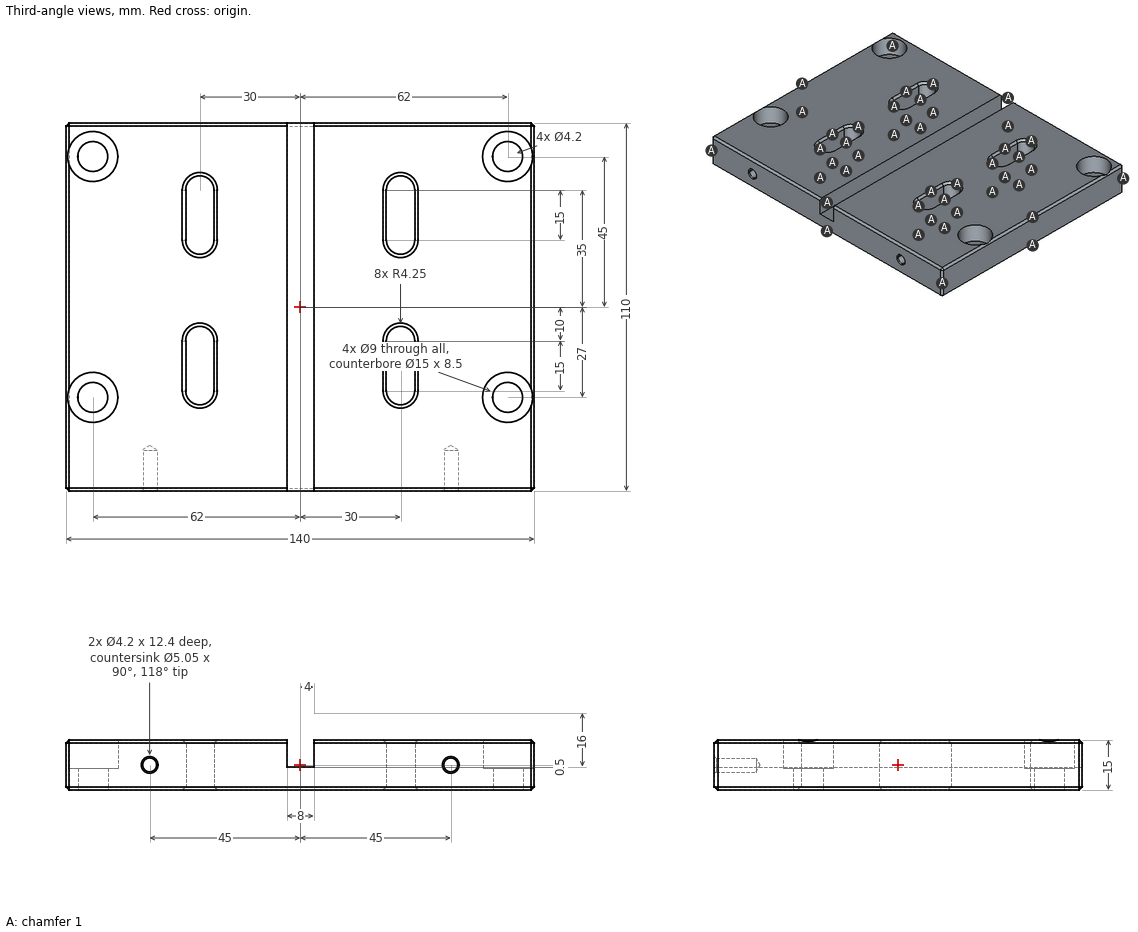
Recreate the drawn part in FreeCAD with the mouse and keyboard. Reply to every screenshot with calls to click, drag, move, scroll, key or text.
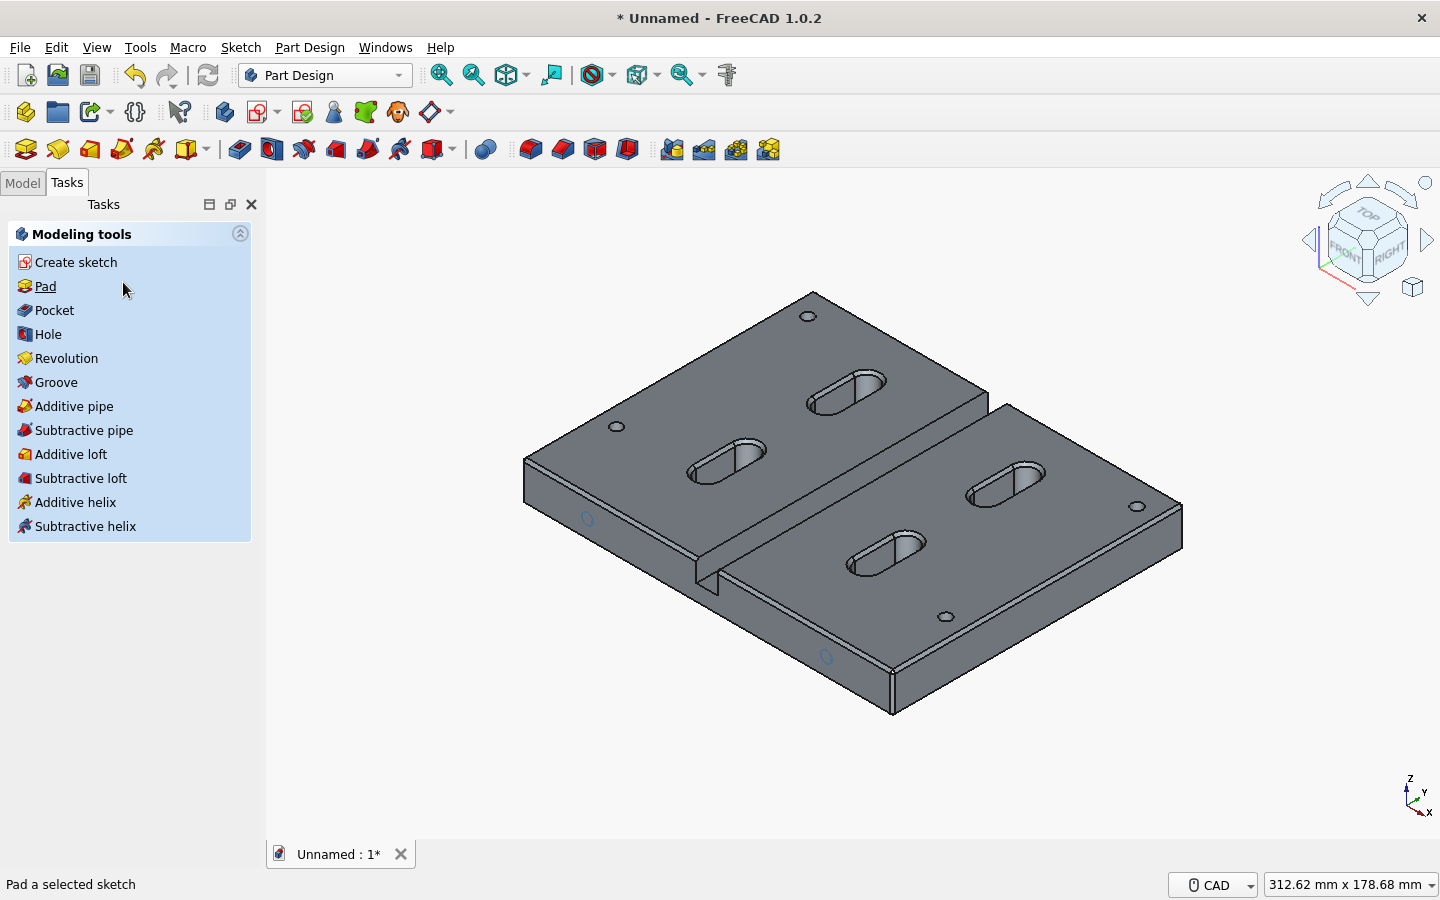
click(272, 150)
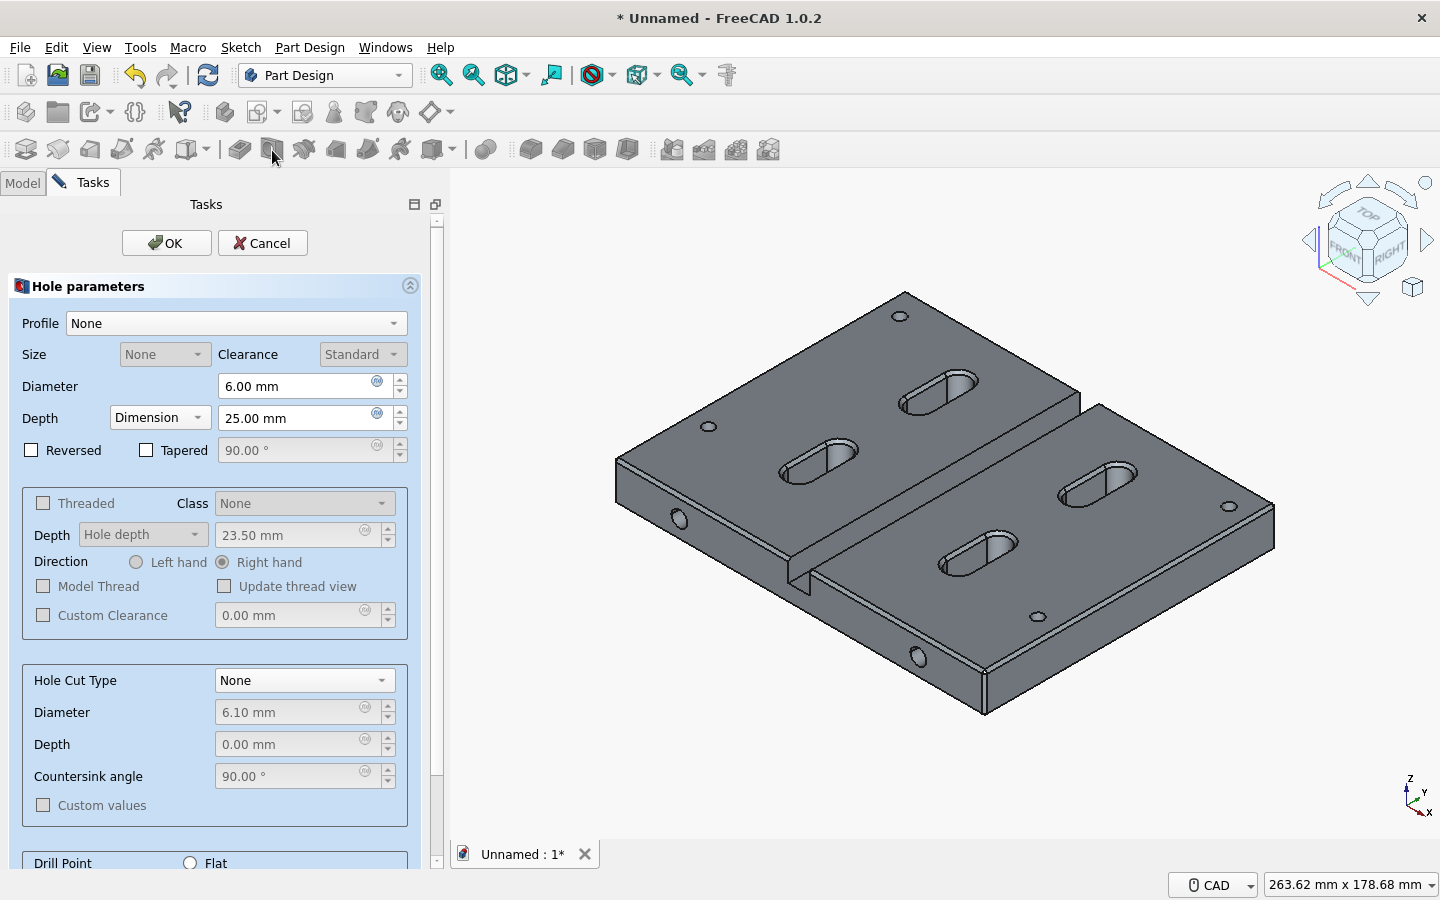
triple_click(305, 386)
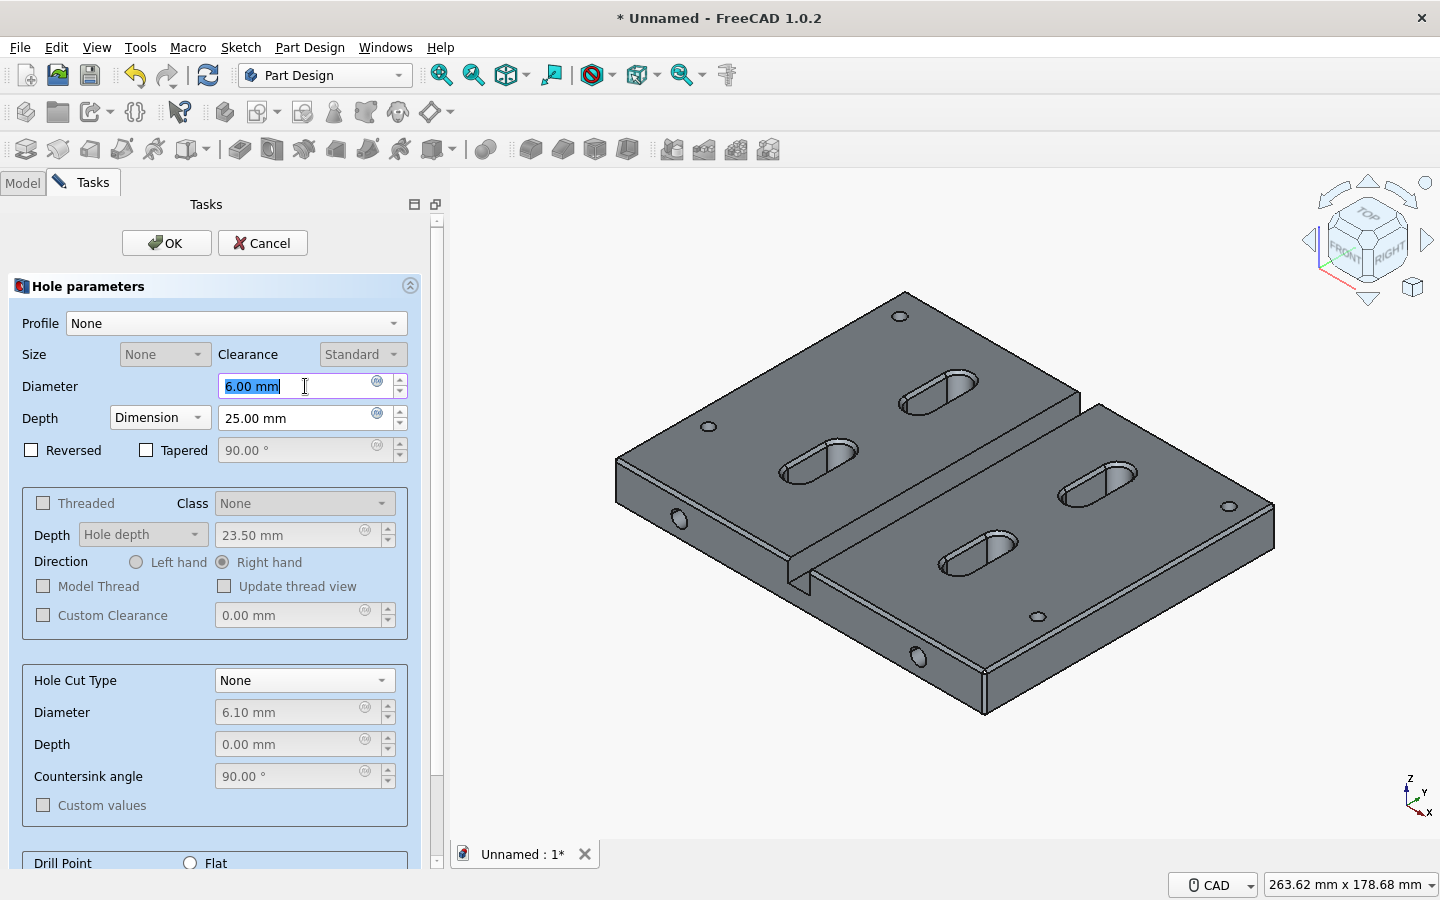
text(4.2)
key(Tab)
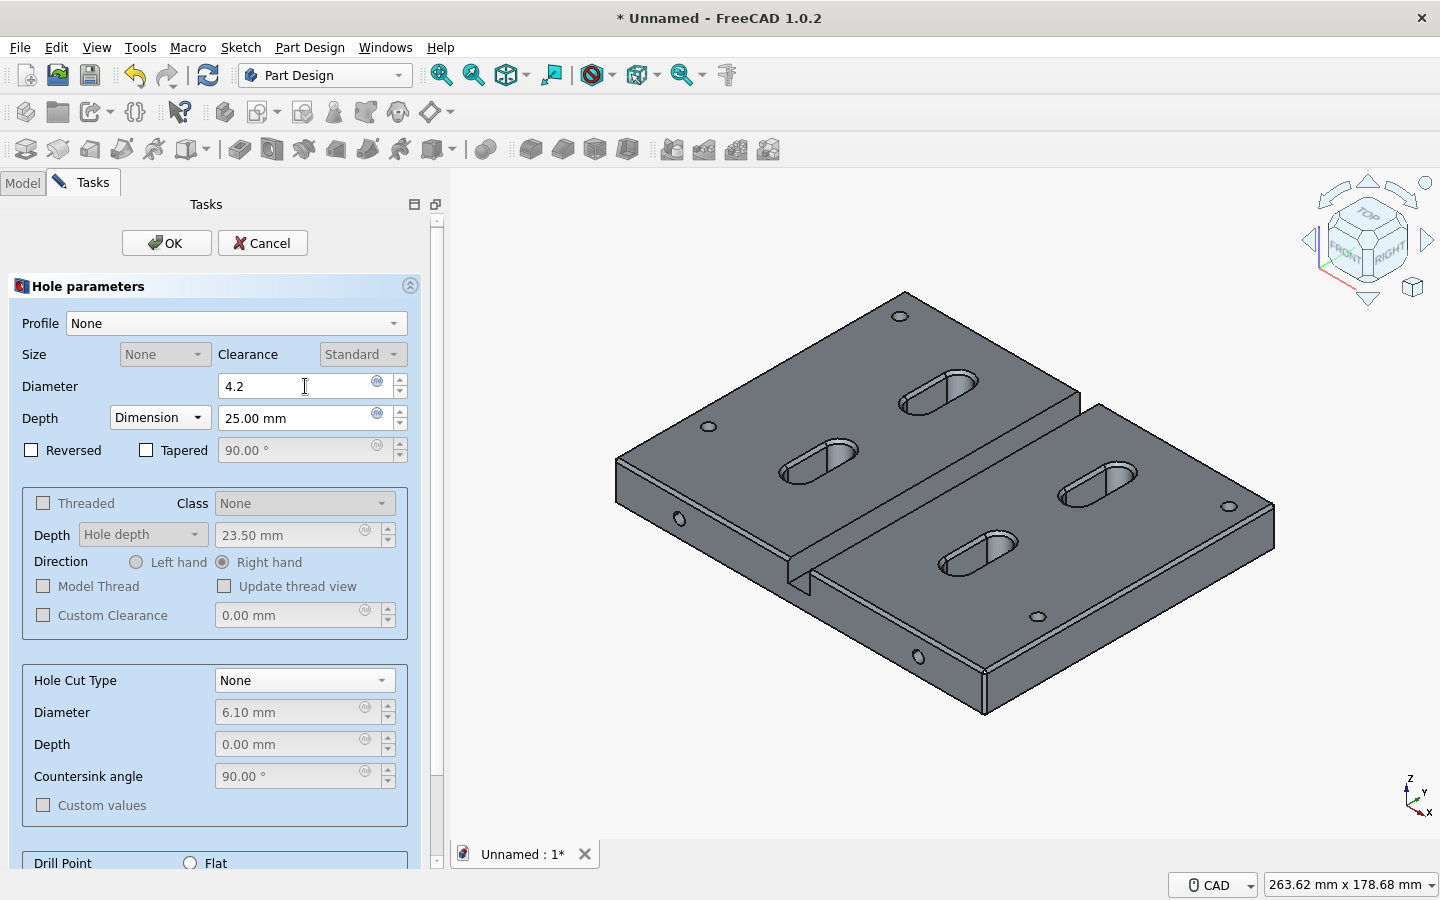
triple_click(305, 418)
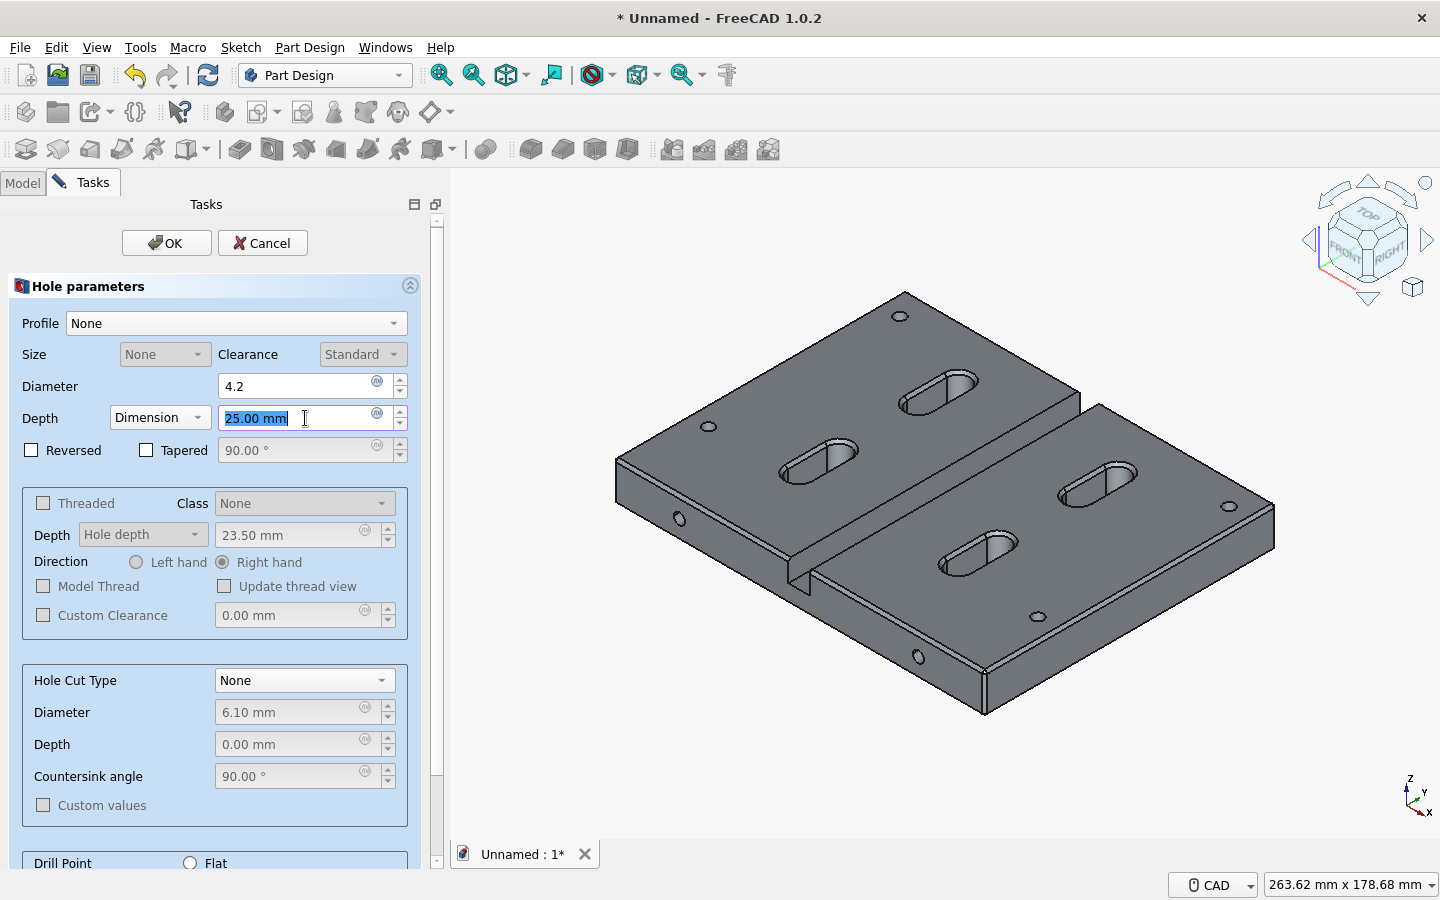
text(12.4)
key(Tab)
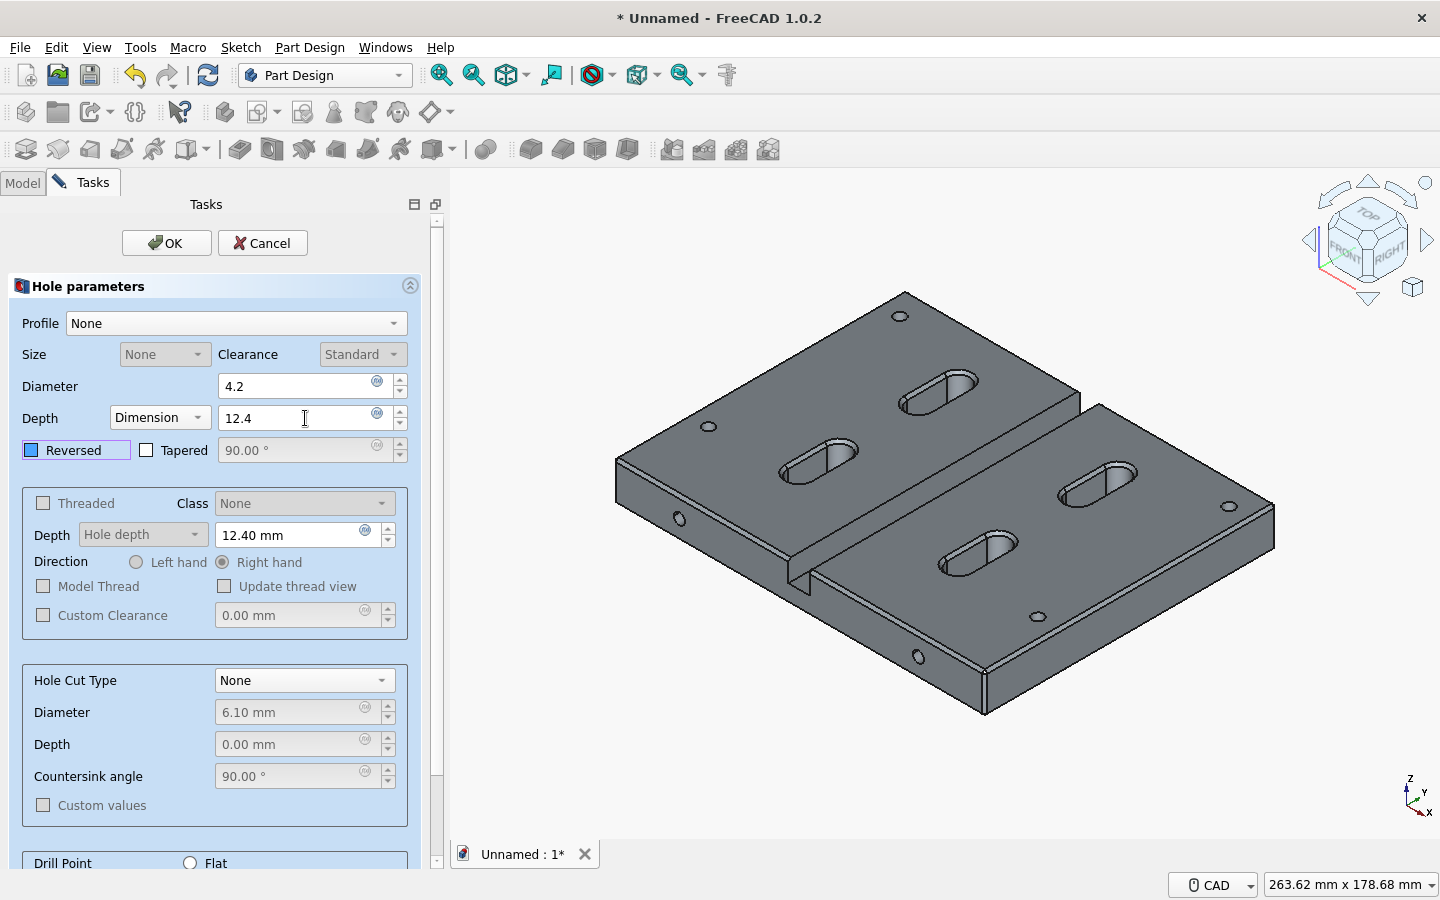
click(306, 680)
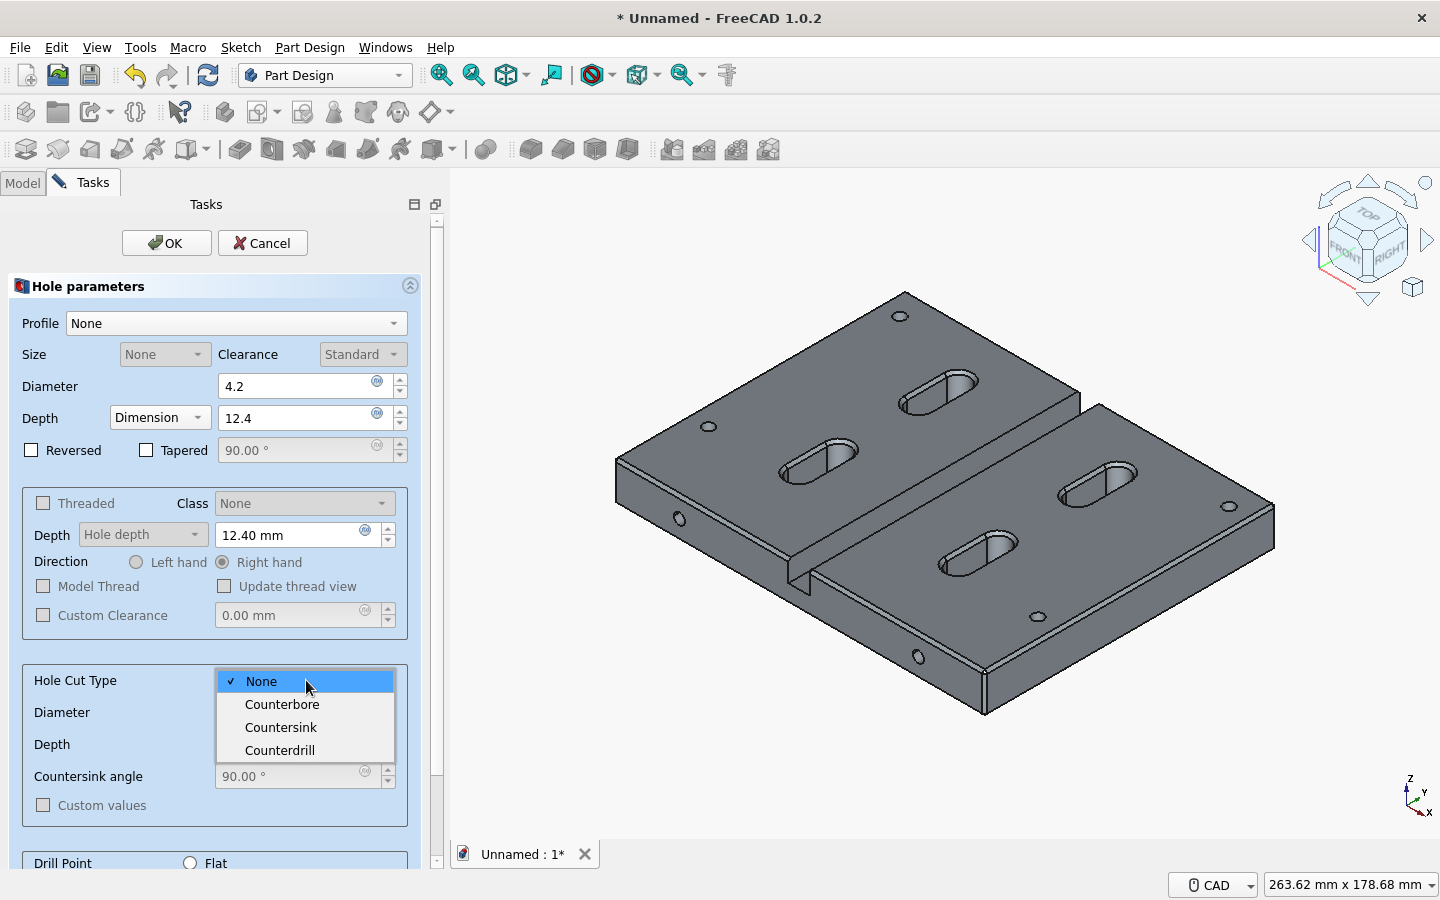
click(304, 728)